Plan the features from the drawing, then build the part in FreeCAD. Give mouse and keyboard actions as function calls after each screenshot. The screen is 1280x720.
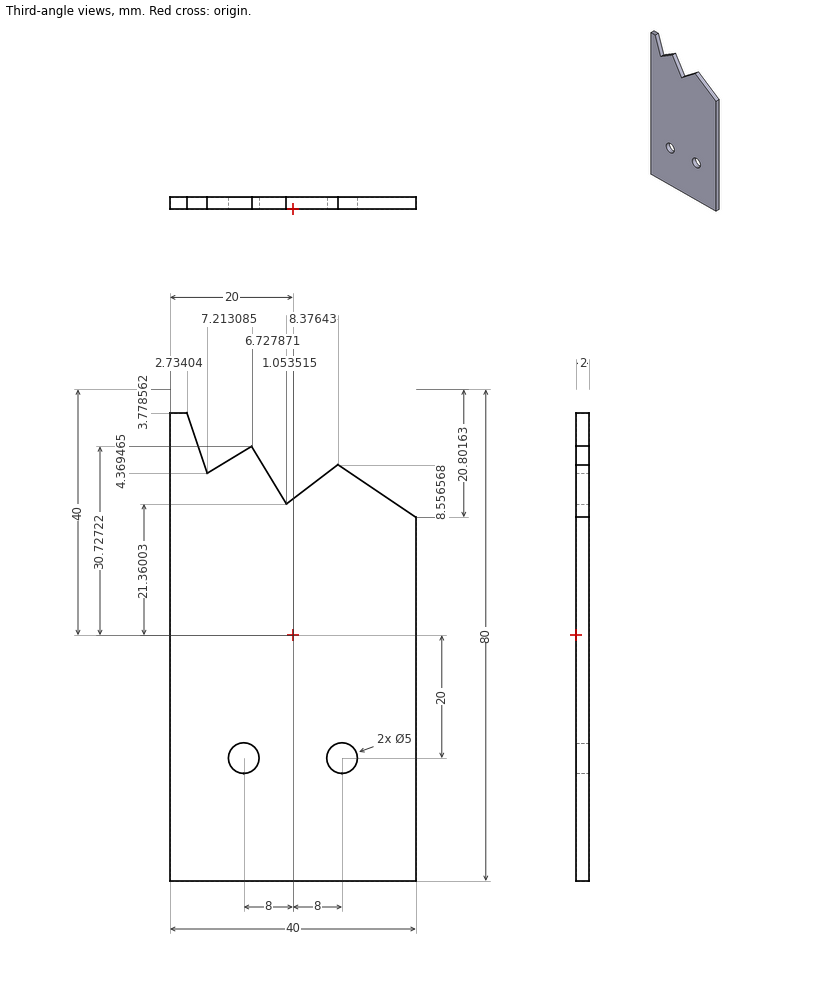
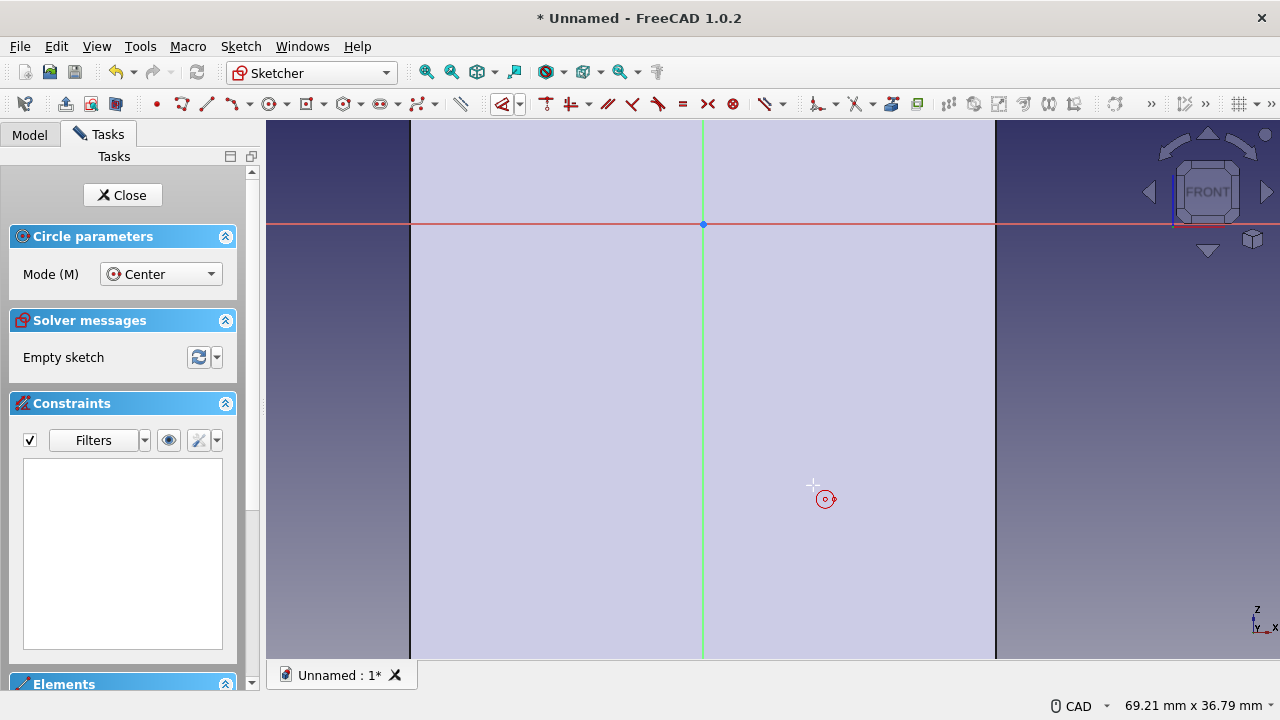
click(821, 517)
click(846, 491)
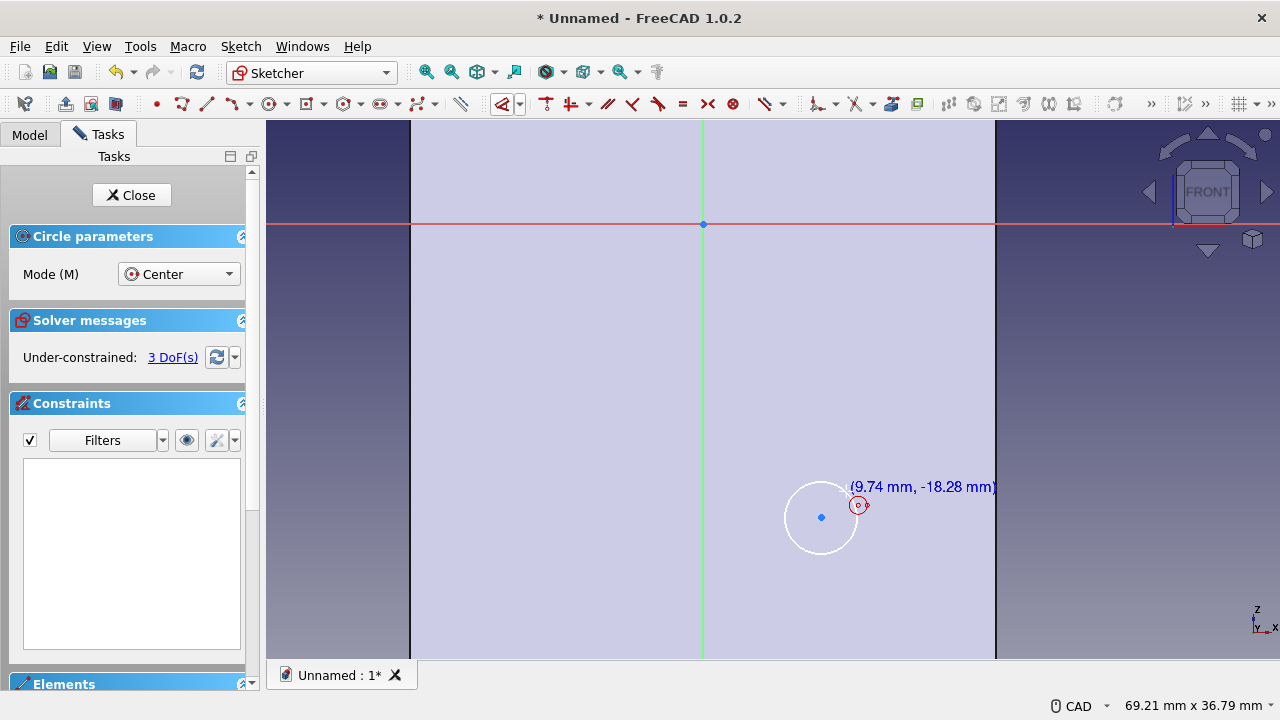
click(586, 517)
click(612, 491)
key(Escape)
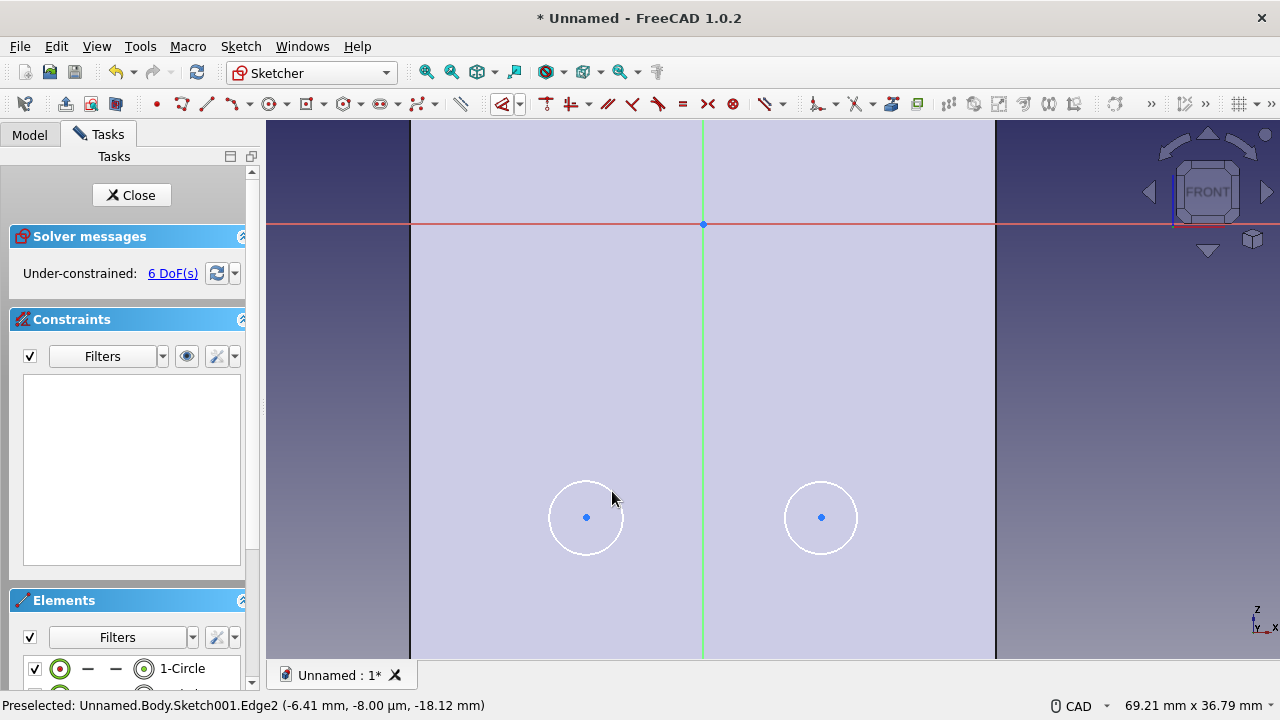
click(846, 492)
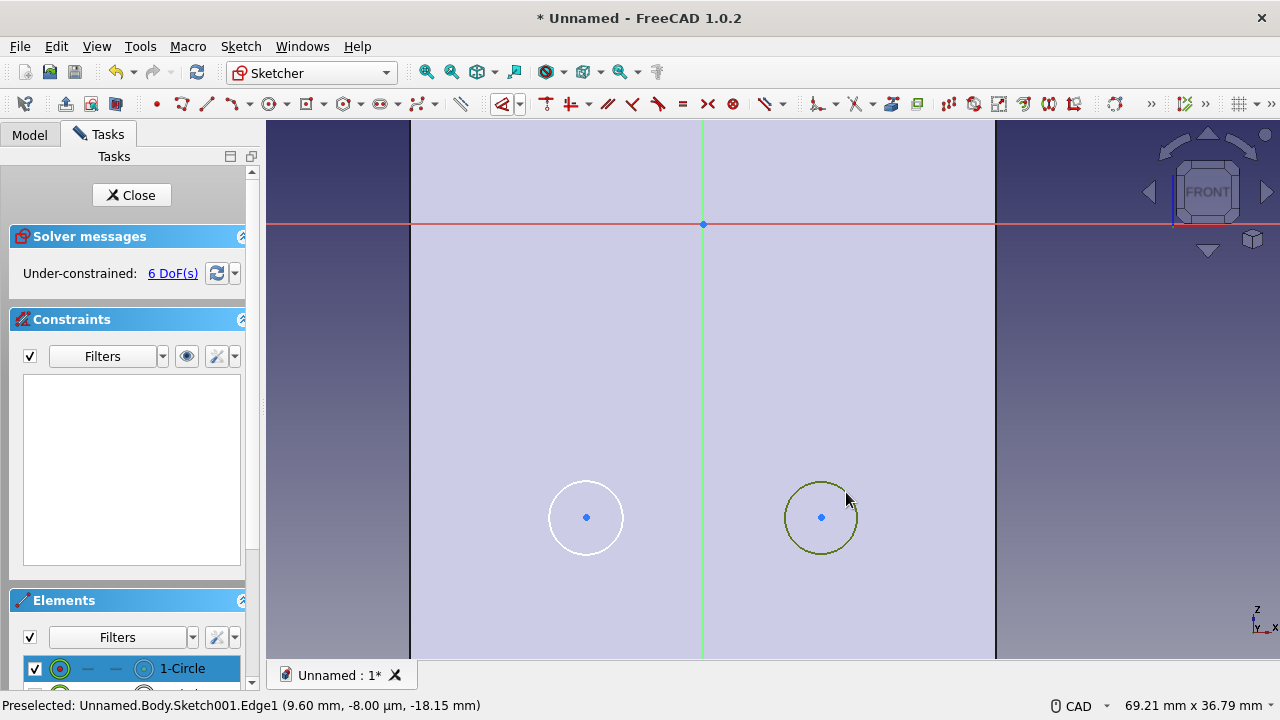
click(612, 492)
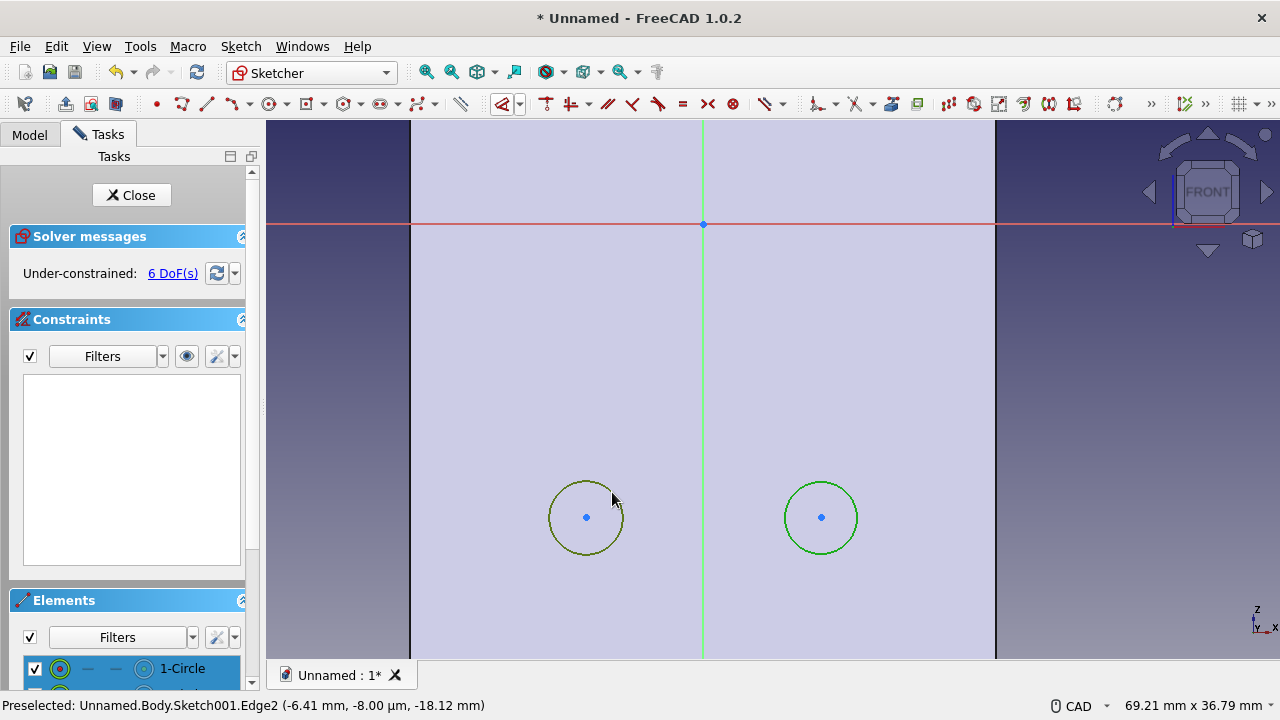
key(e)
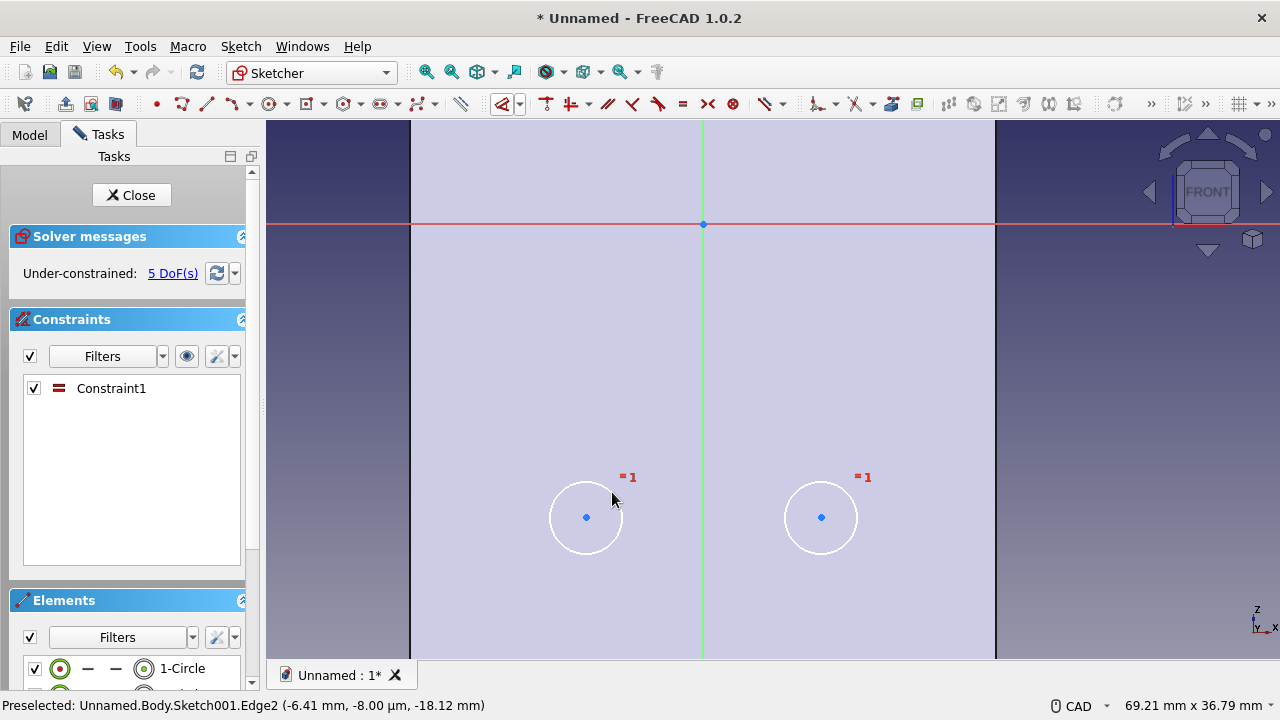
click(821, 518)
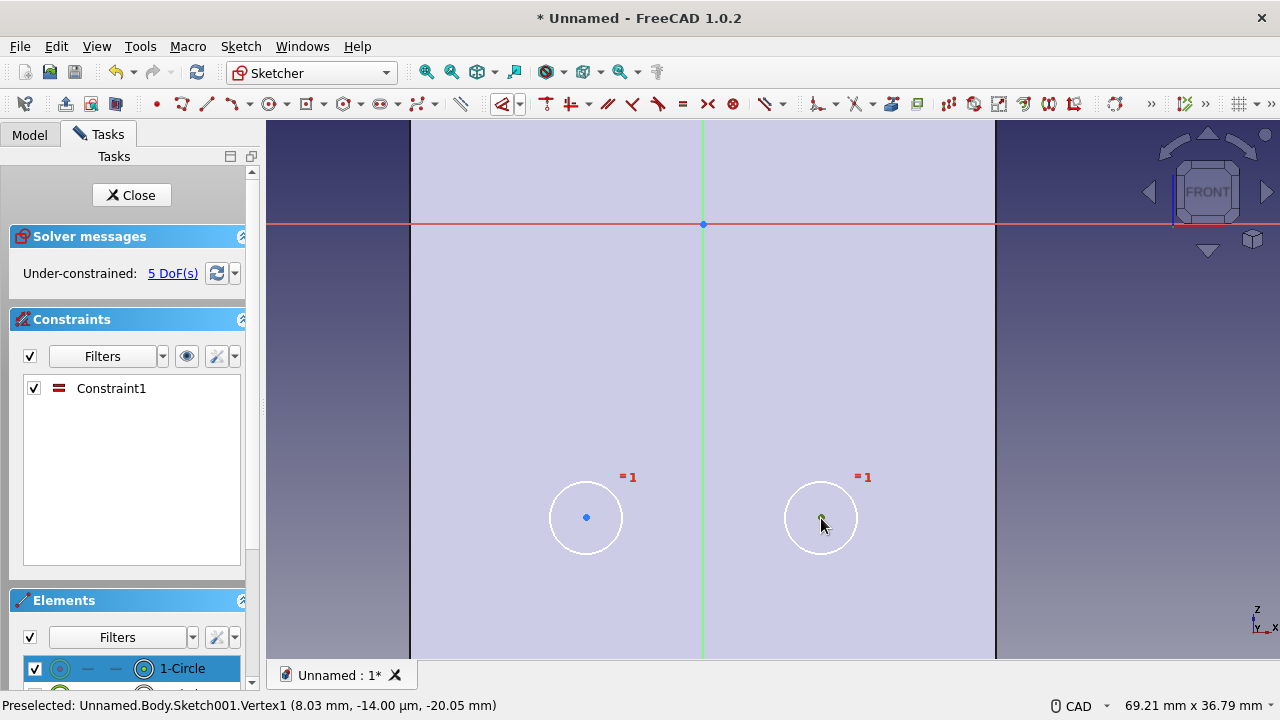
click(586, 518)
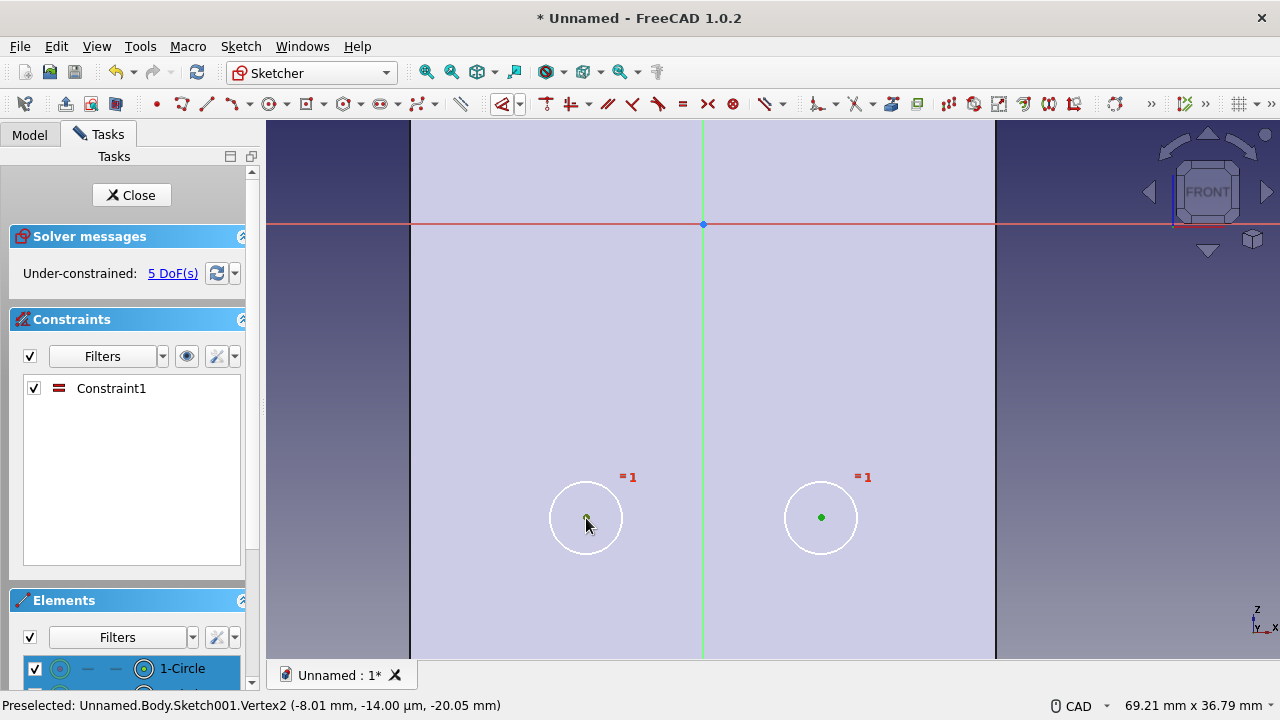
click(588, 104)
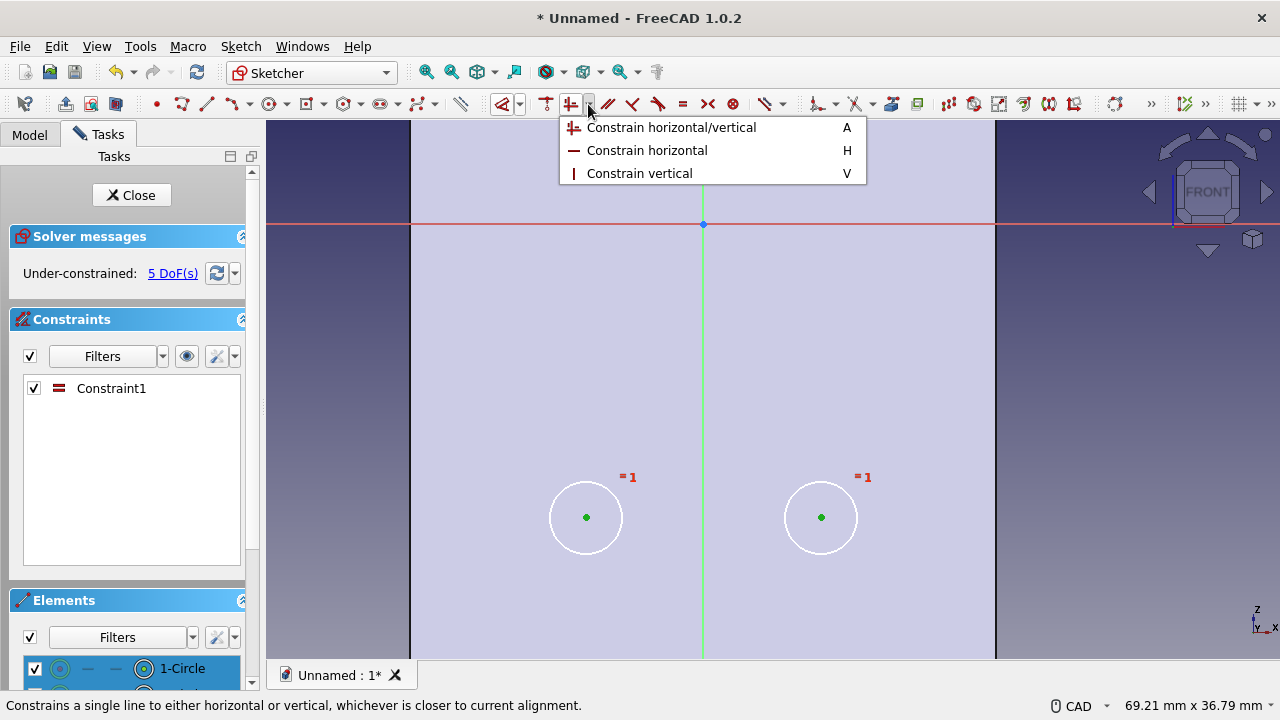
click(713, 150)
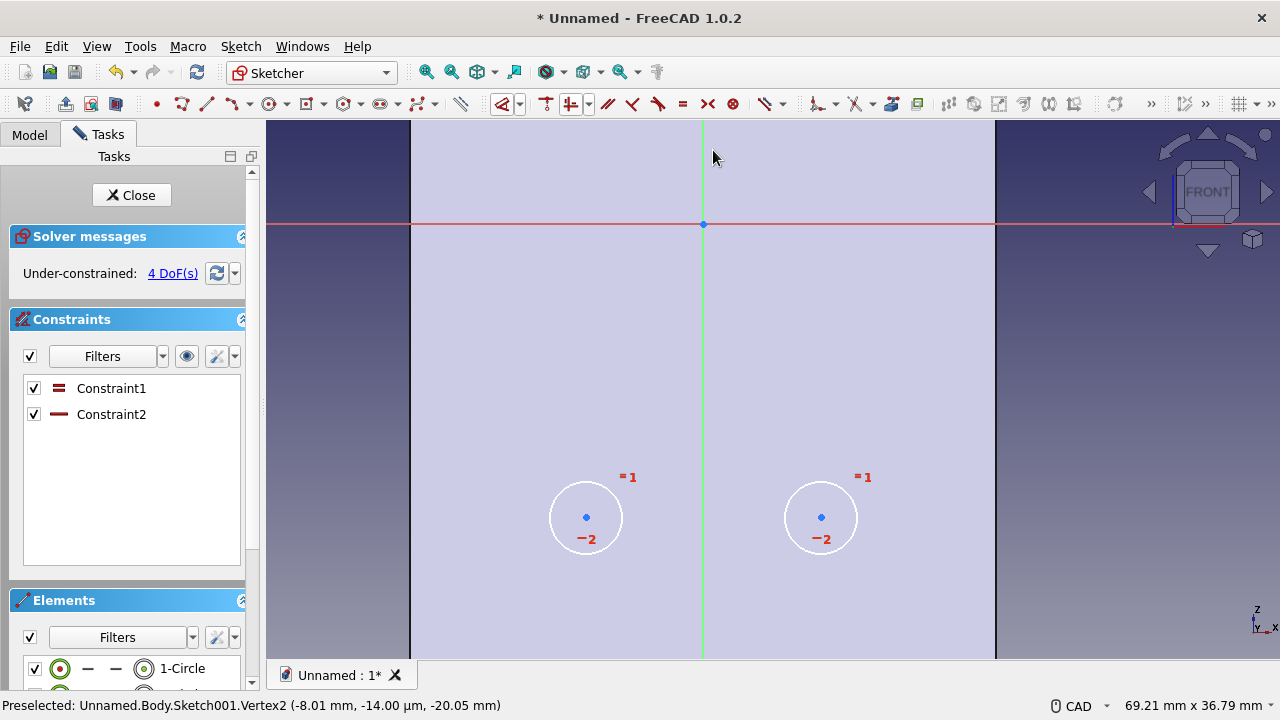
click(846, 492)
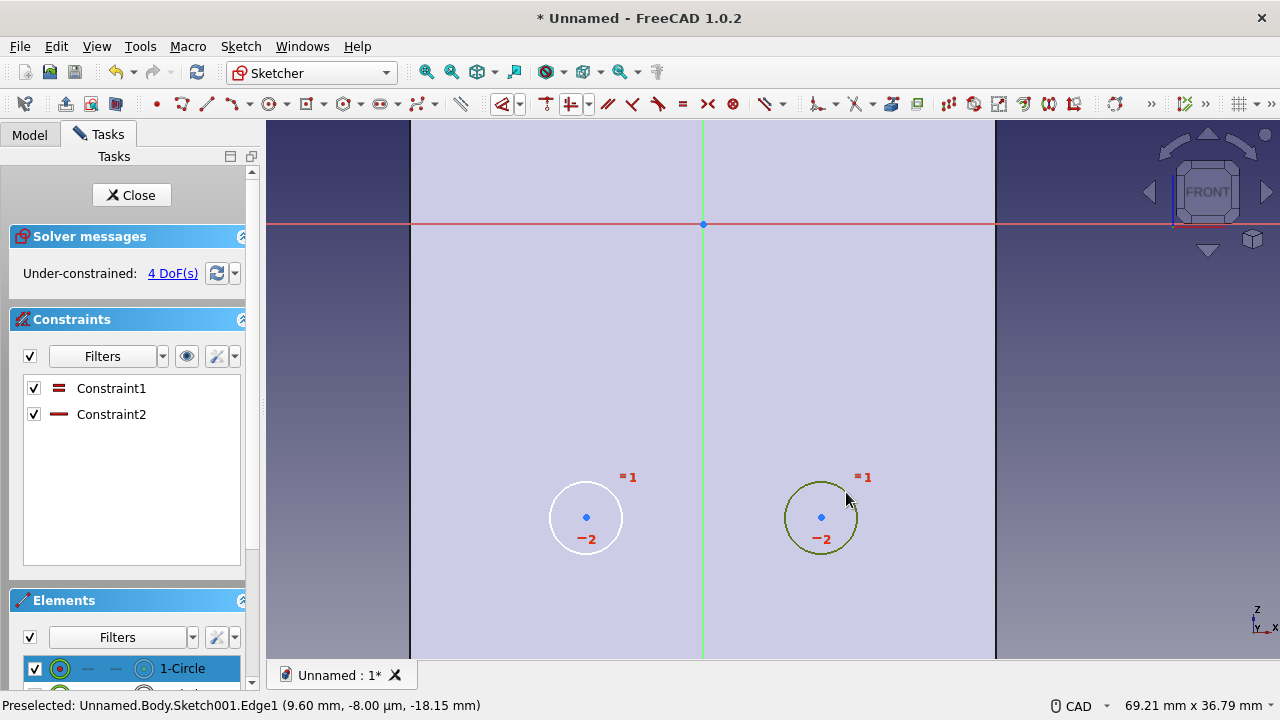
key(k)
key(o)